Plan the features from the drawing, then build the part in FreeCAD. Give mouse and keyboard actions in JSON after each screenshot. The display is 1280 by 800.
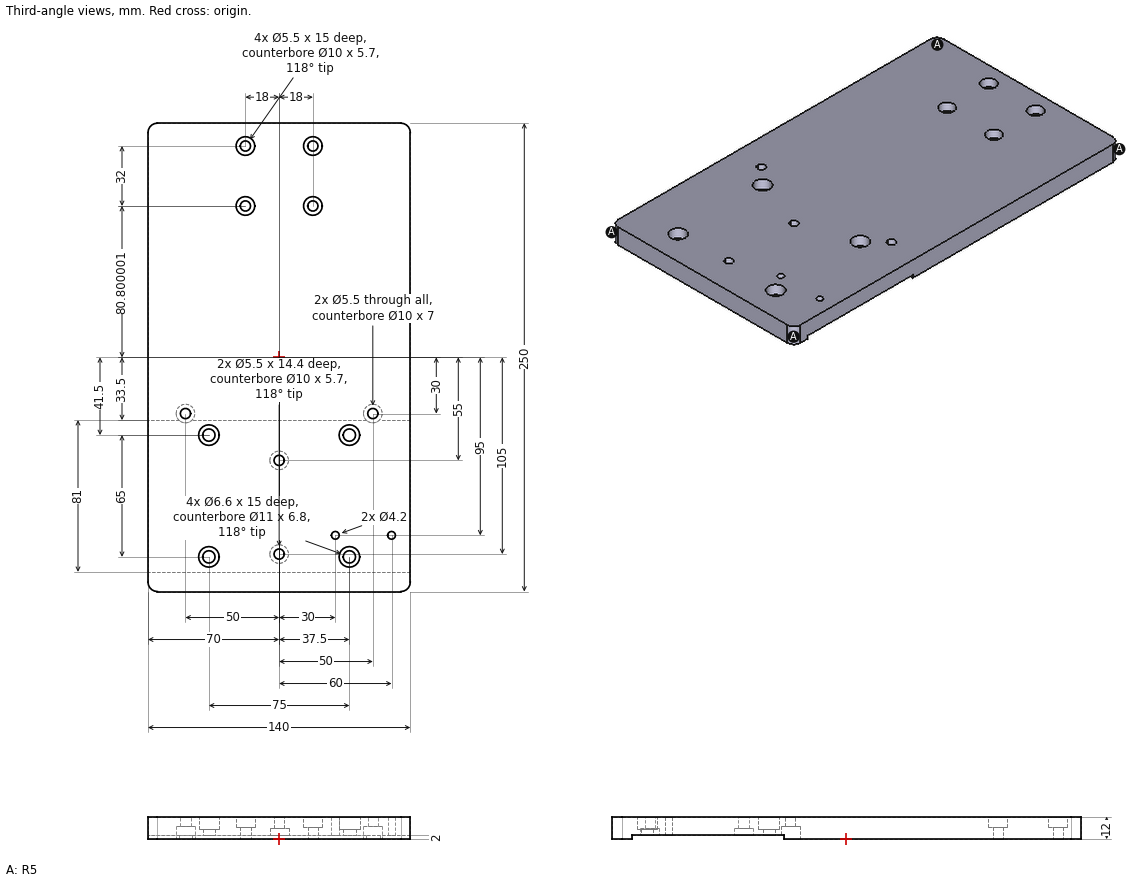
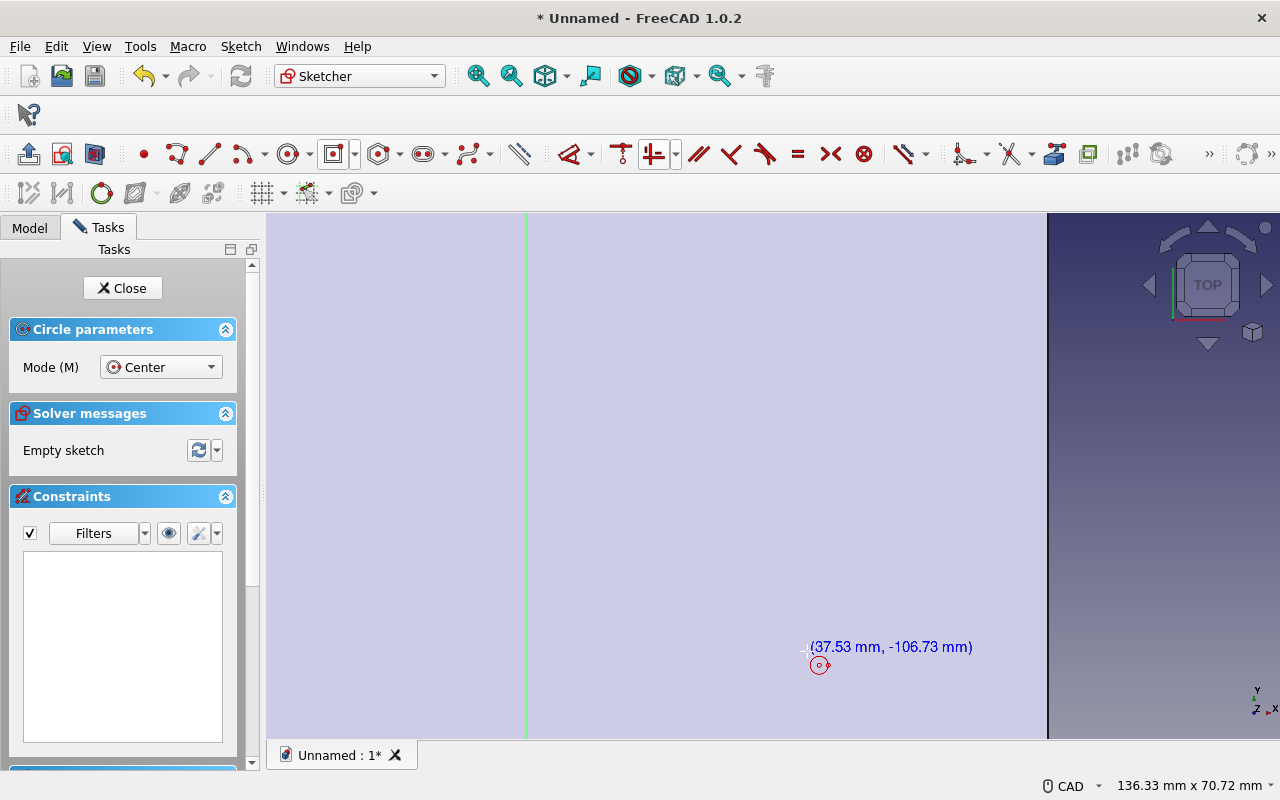
{"action": "left_click", "coordinate": [806, 651]}
{"action": "left_click", "coordinate": [823, 633]}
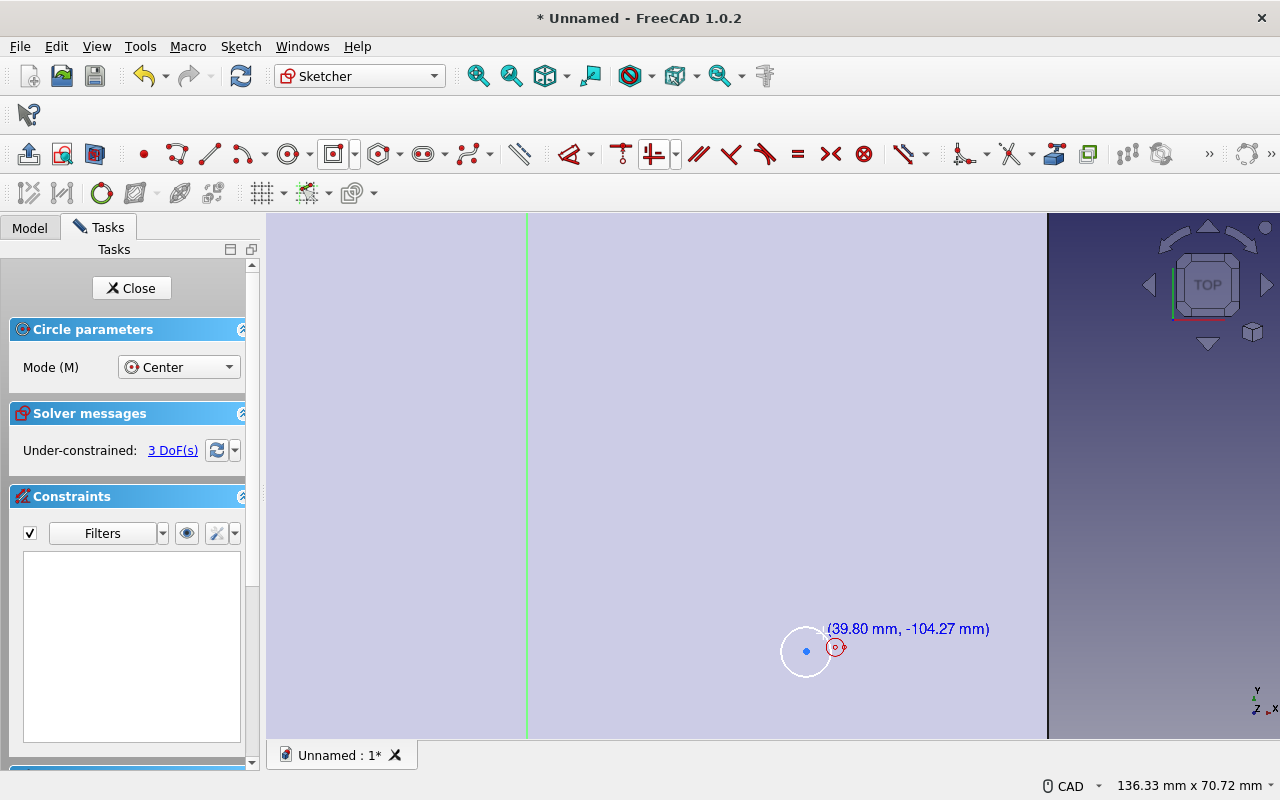
{"action": "scroll", "coordinate": [808, 598], "scroll_direction": "down", "scroll_amount": 5}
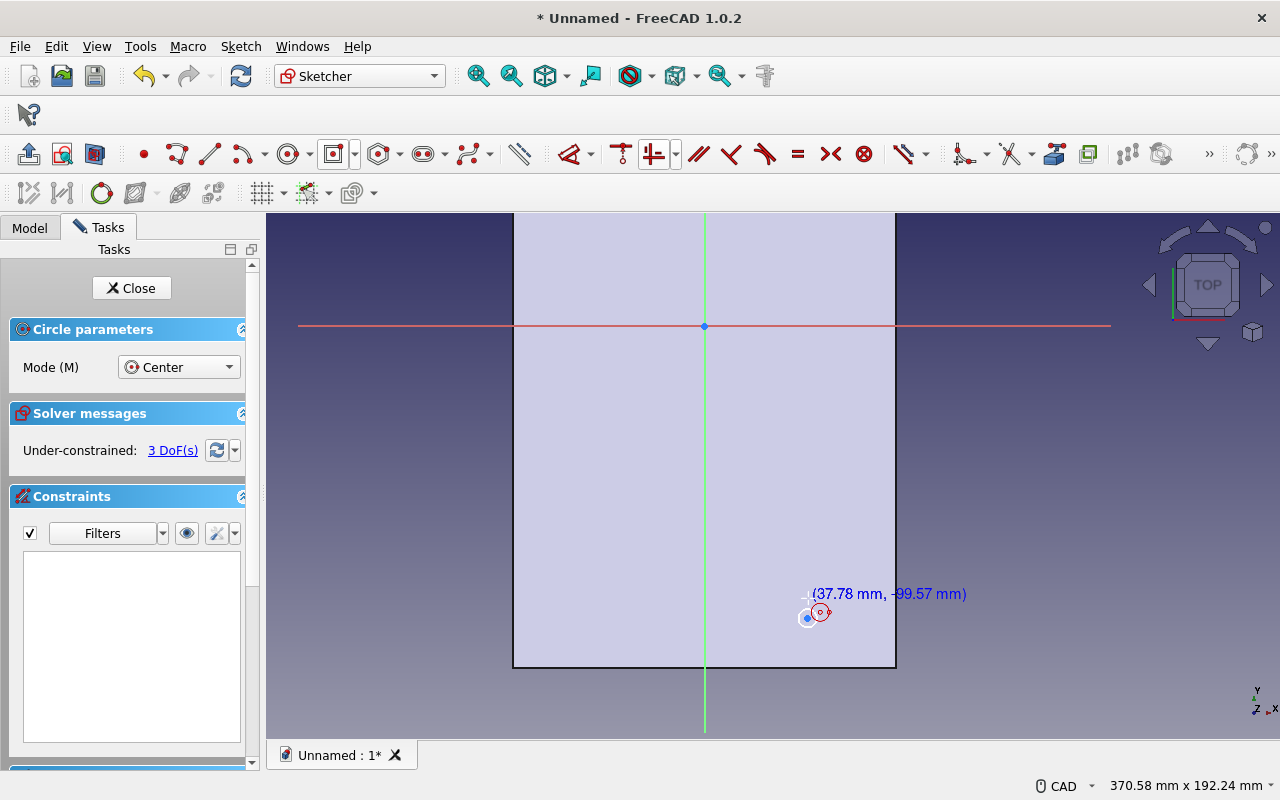
{"action": "scroll", "coordinate": [602, 618], "scroll_direction": "up", "scroll_amount": 5}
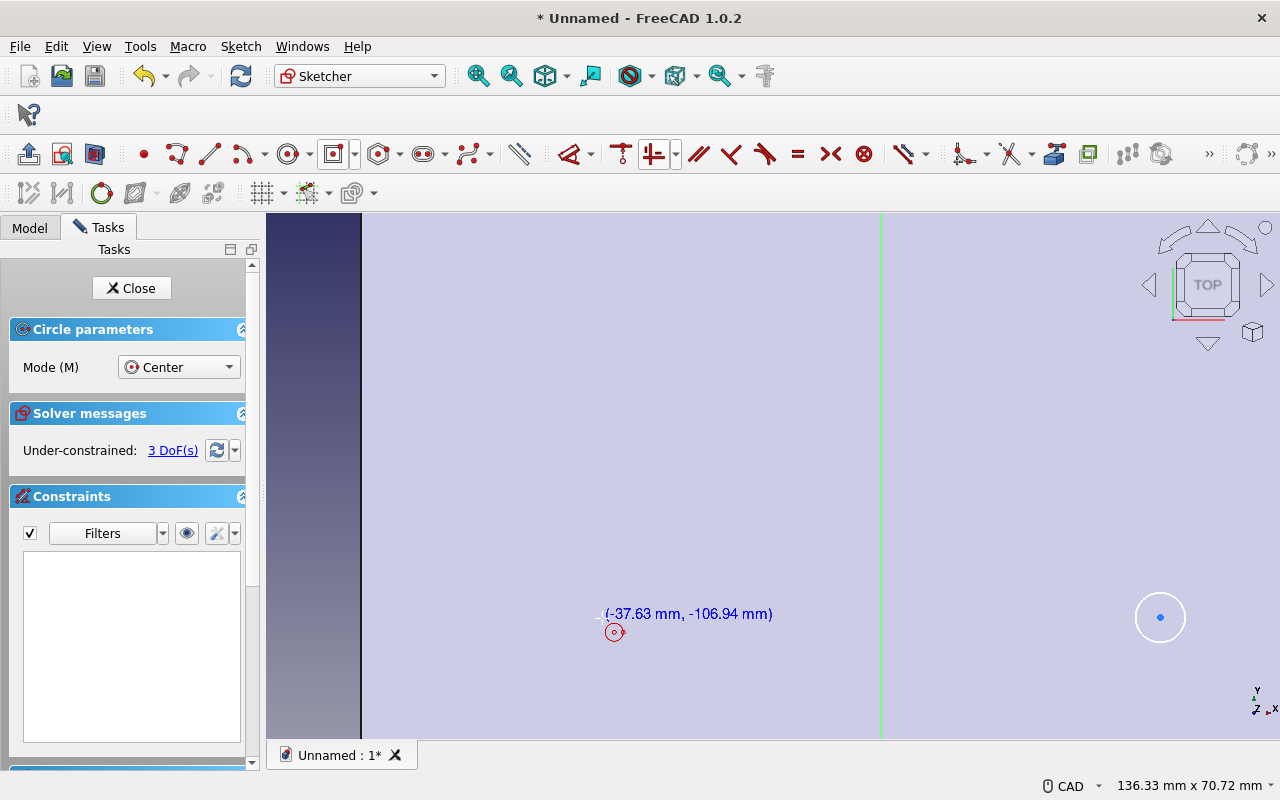
{"action": "left_click", "coordinate": [602, 616]}
{"action": "left_click", "coordinate": [620, 599]}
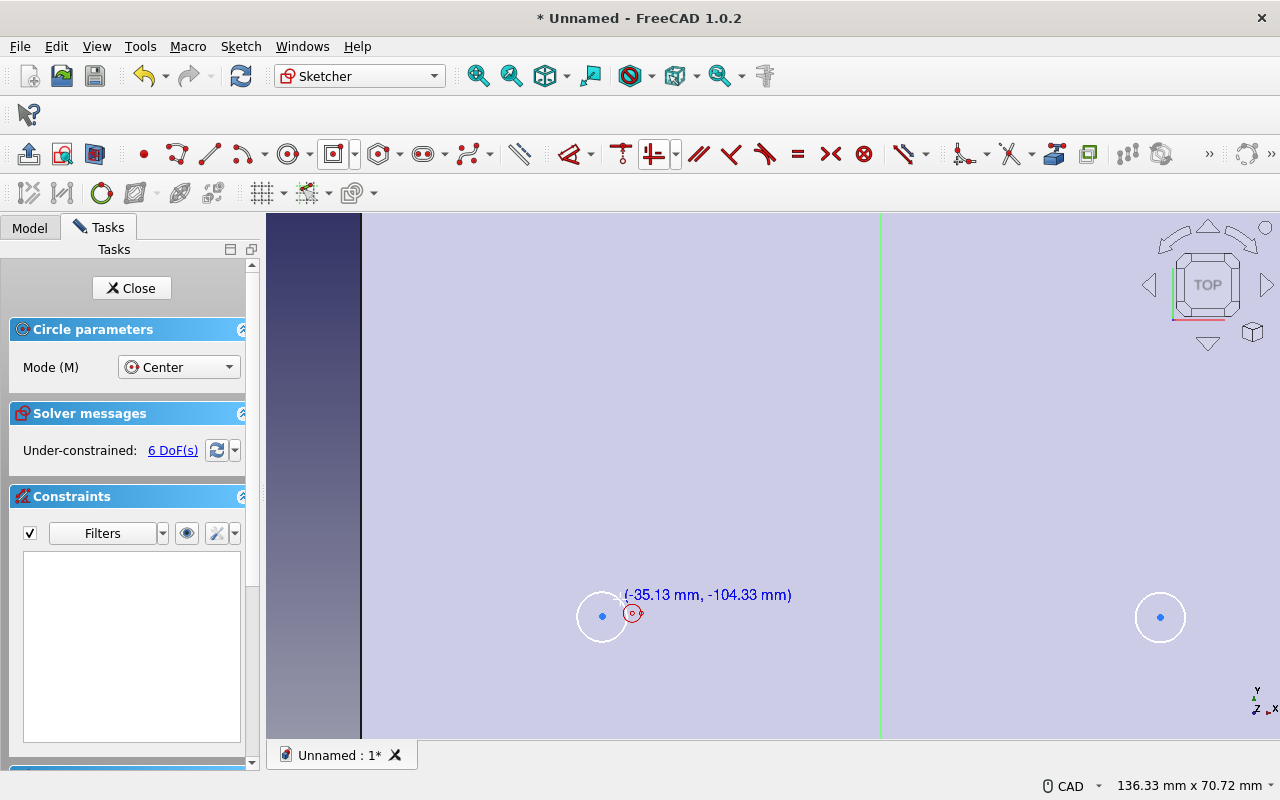
{"action": "scroll", "coordinate": [602, 618], "scroll_direction": "down", "scroll_amount": 5}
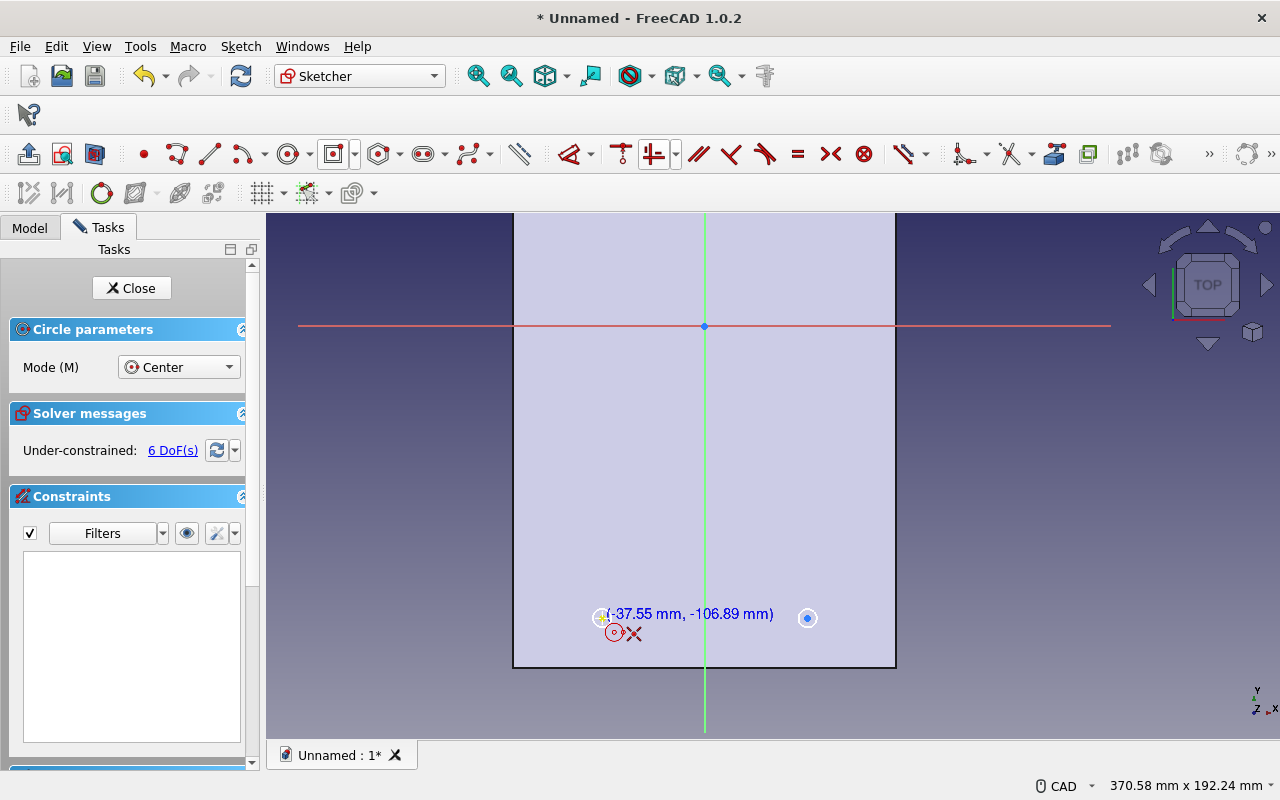
{"action": "scroll", "coordinate": [602, 440], "scroll_direction": "up", "scroll_amount": 5}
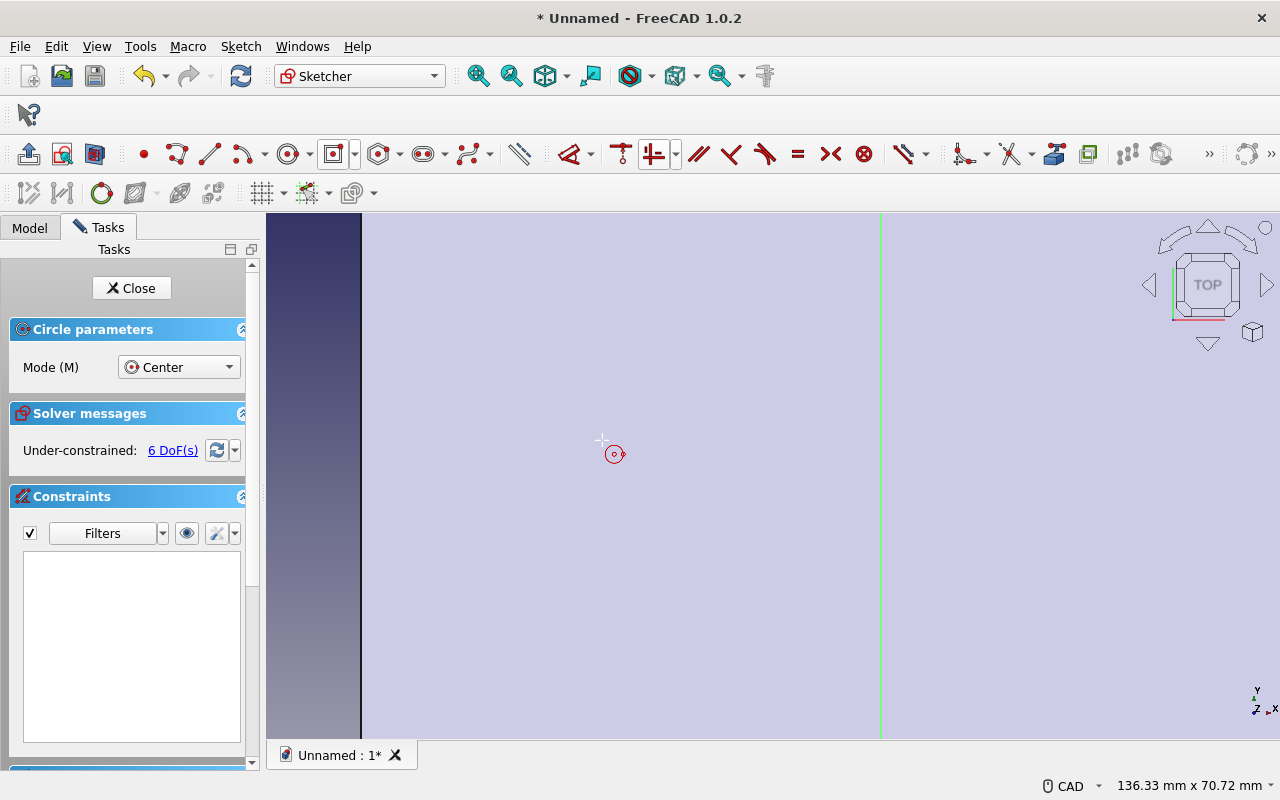
{"action": "left_click", "coordinate": [602, 439]}
{"action": "left_click", "coordinate": [620, 422]}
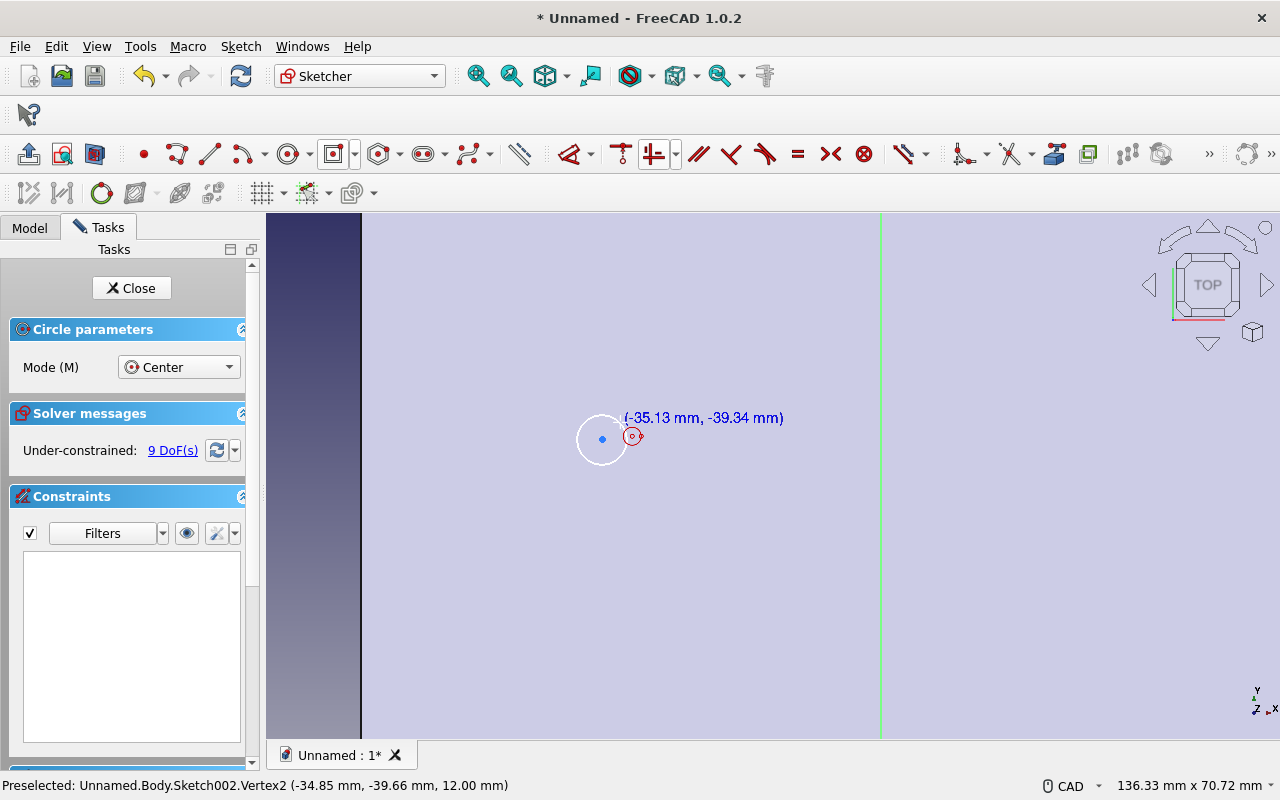
{"action": "scroll", "coordinate": [602, 439], "scroll_direction": "down", "scroll_amount": 5}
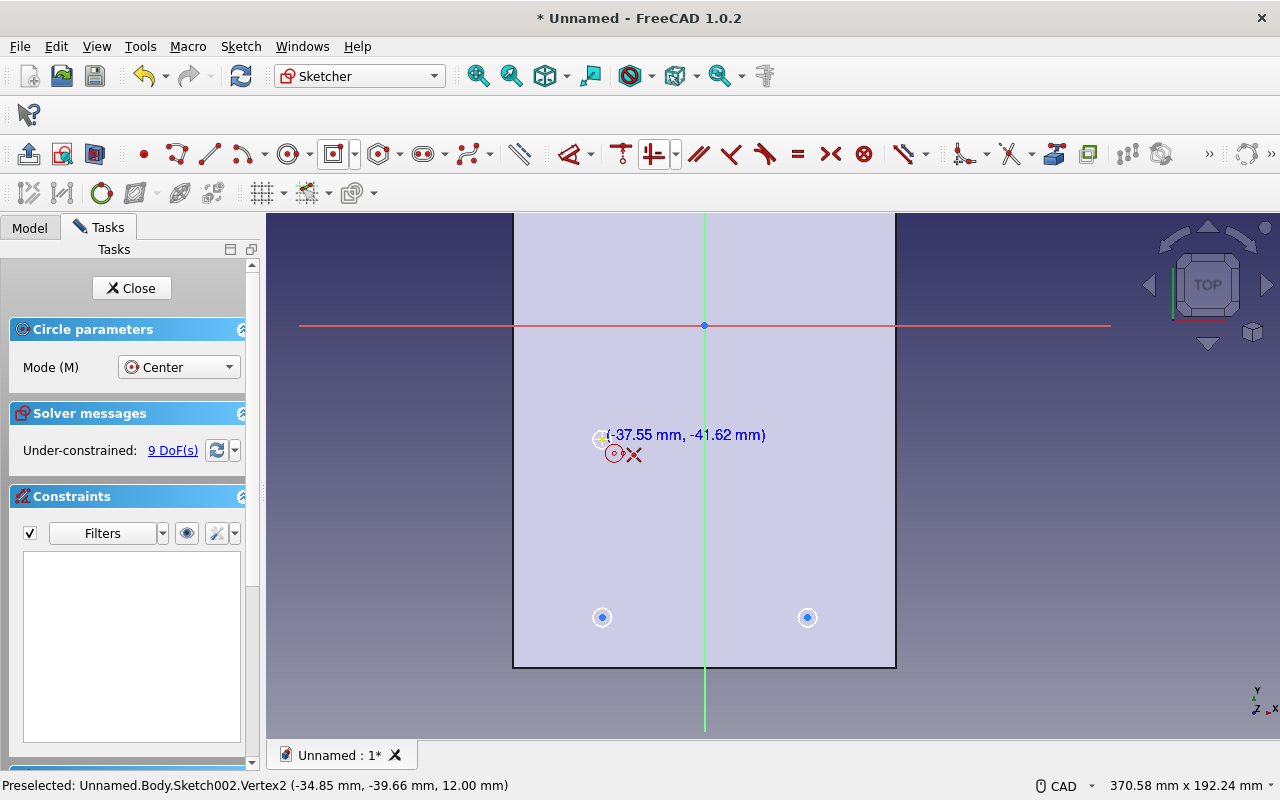
{"action": "scroll", "coordinate": [808, 439], "scroll_direction": "up", "scroll_amount": 5}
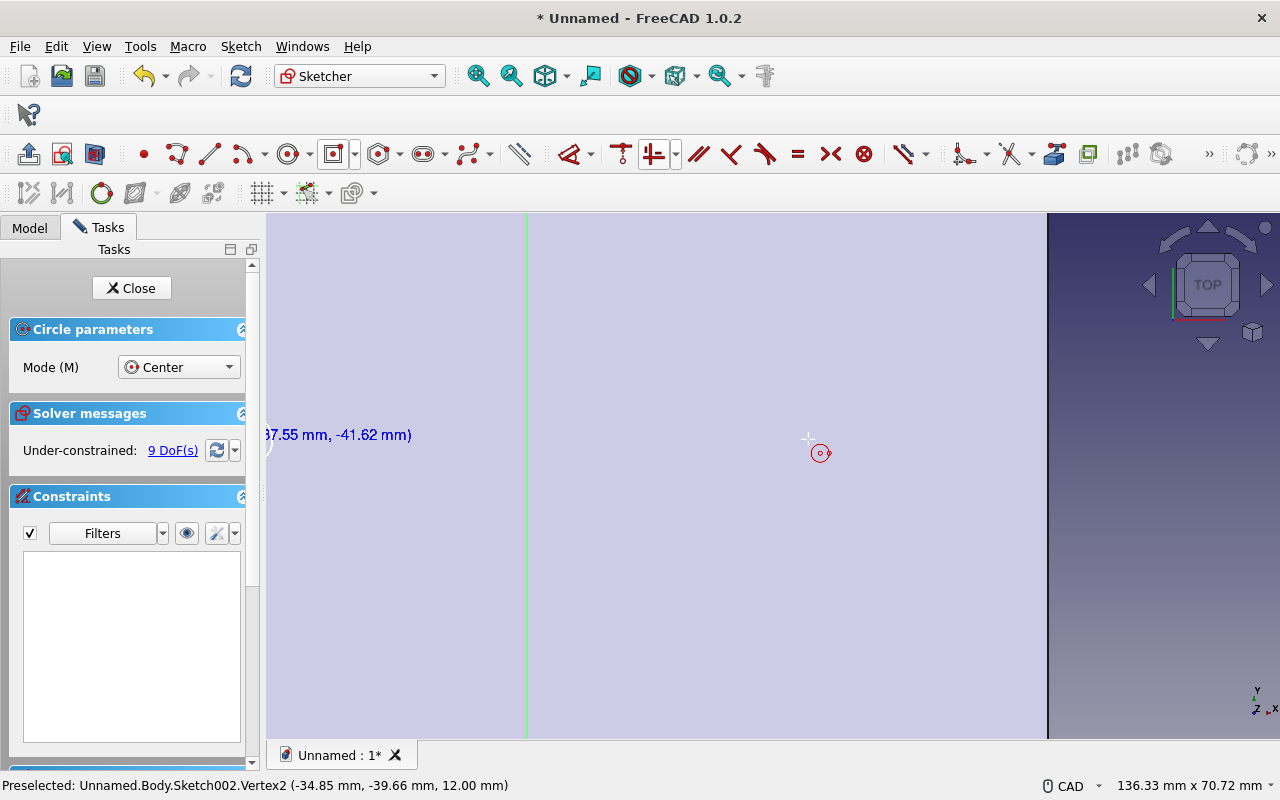
{"action": "left_click", "coordinate": [806, 439]}
{"action": "left_click", "coordinate": [823, 422]}
{"action": "key", "text": "Escape"}